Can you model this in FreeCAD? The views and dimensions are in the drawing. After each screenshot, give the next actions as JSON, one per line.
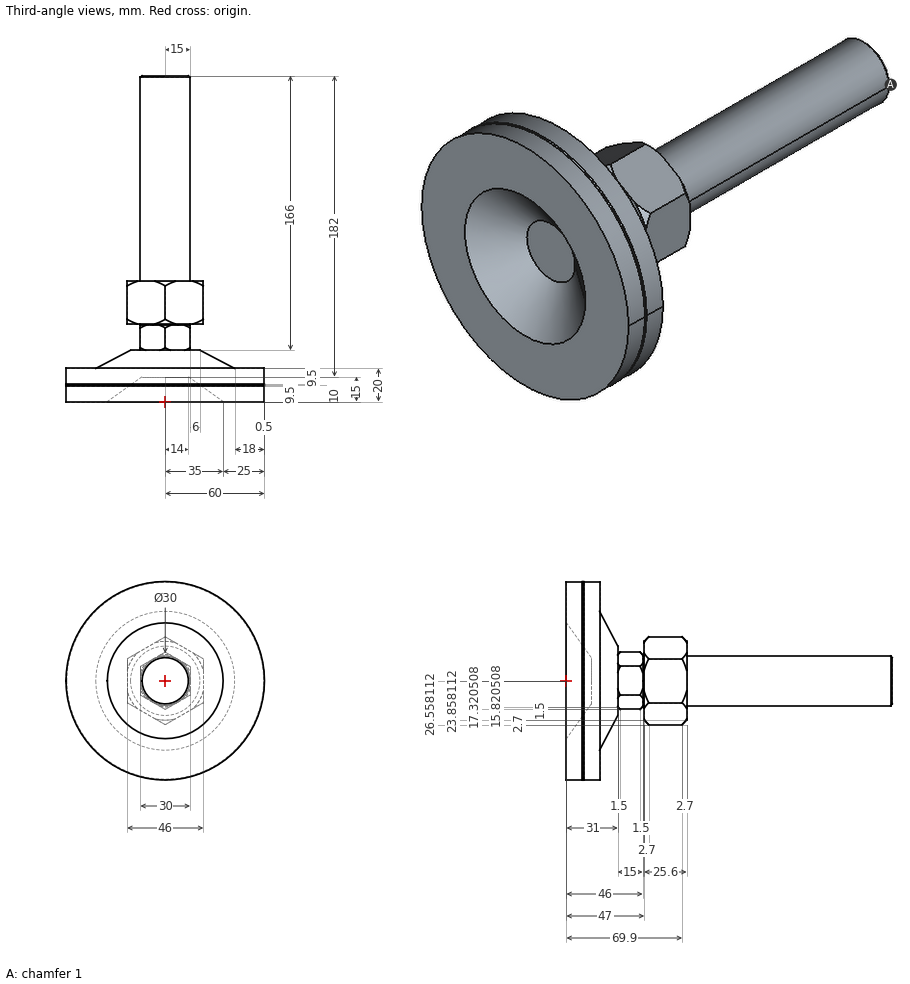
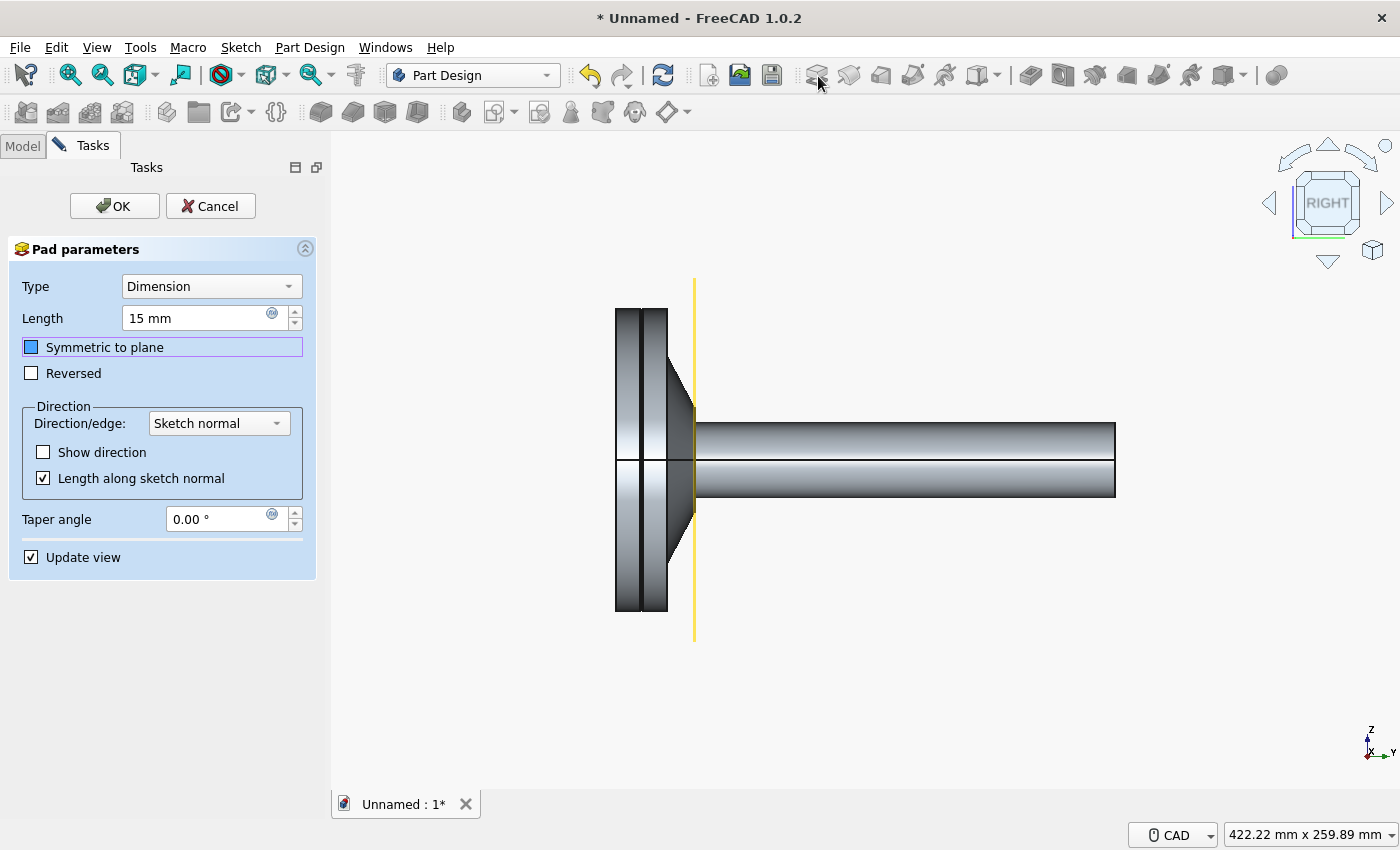
{"action": "left_click", "coordinate": [30, 373]}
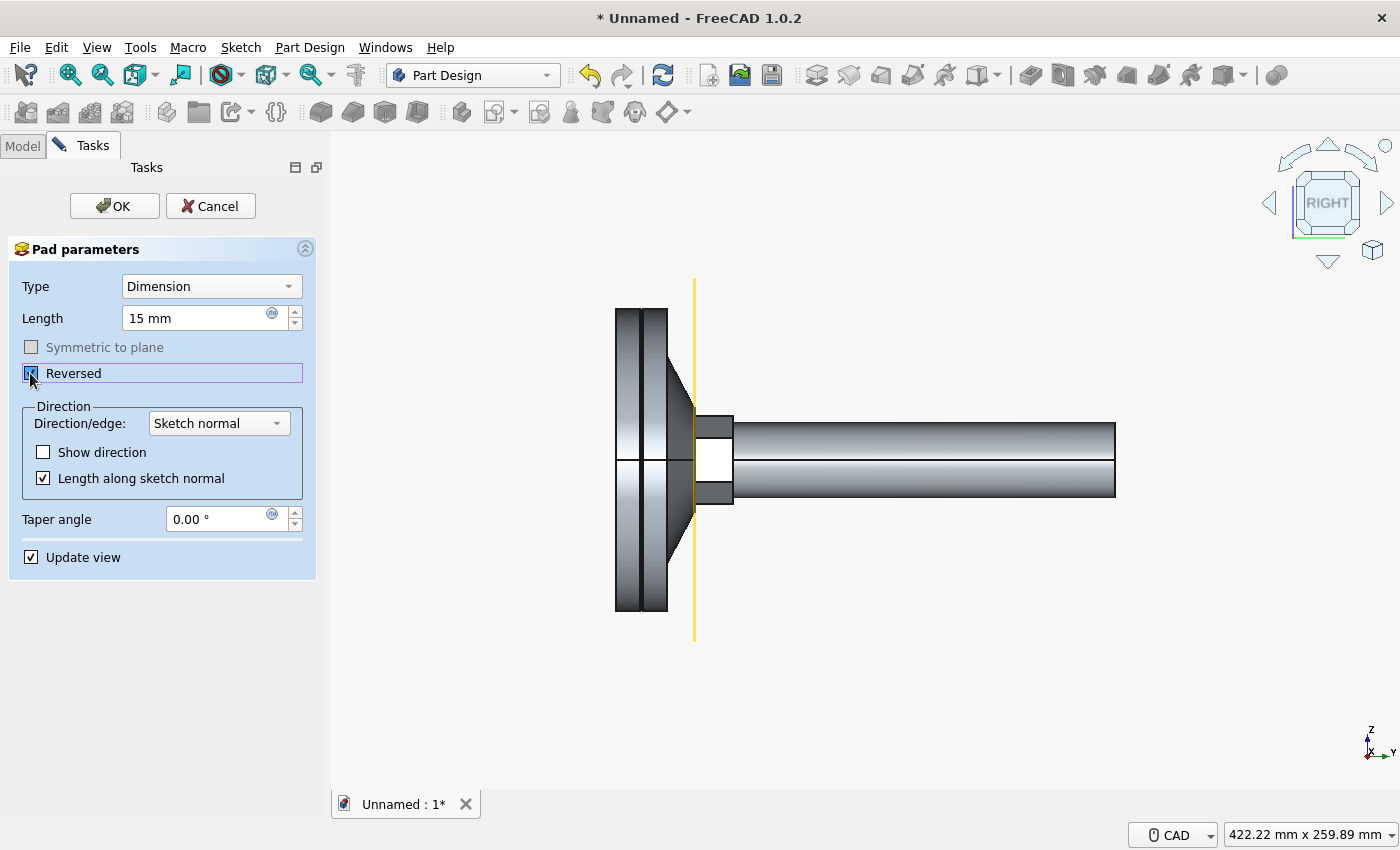
{"action": "left_click", "coordinate": [115, 206]}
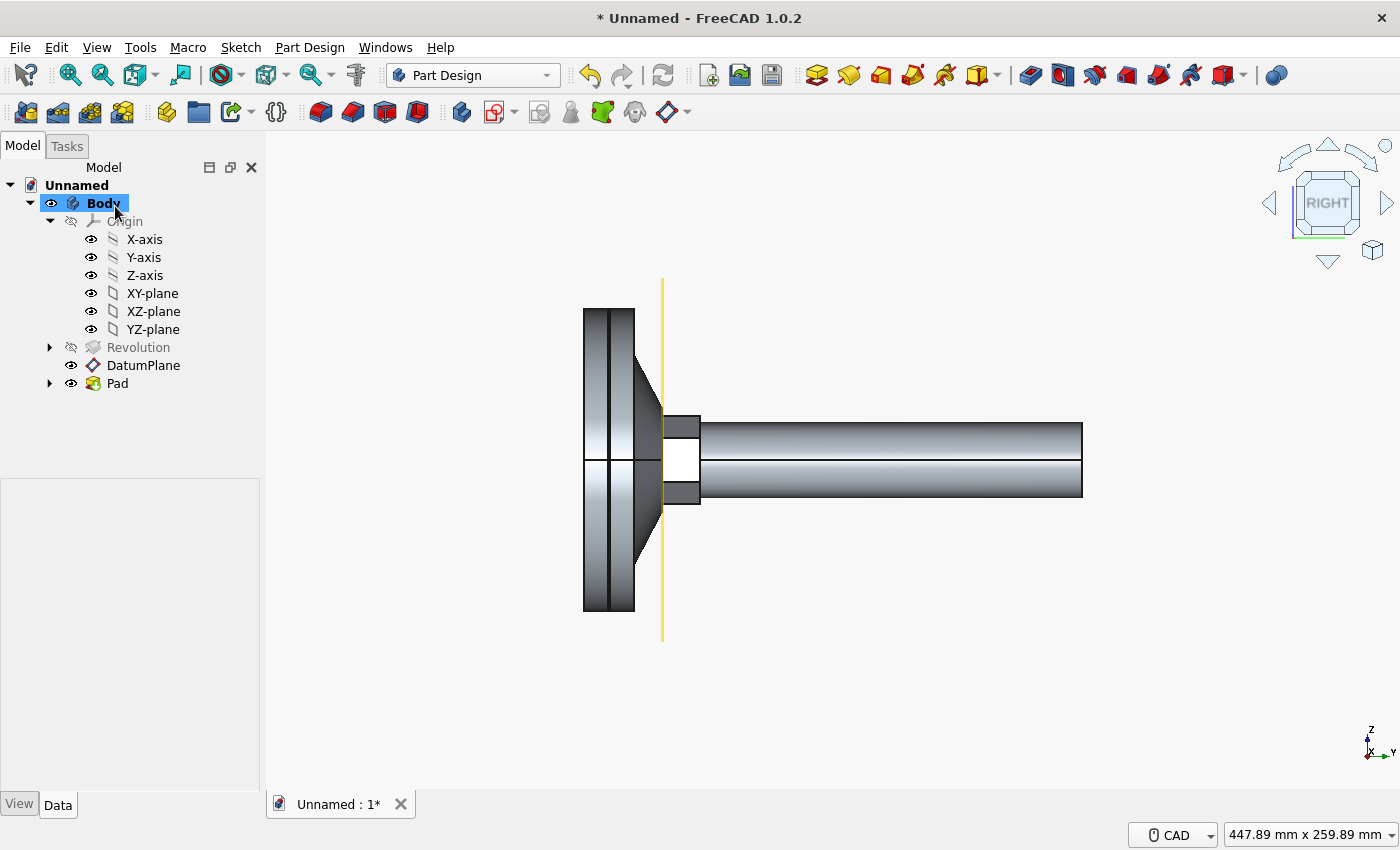
{"action": "left_click", "coordinate": [116, 365]}
{"action": "key", "text": "space"}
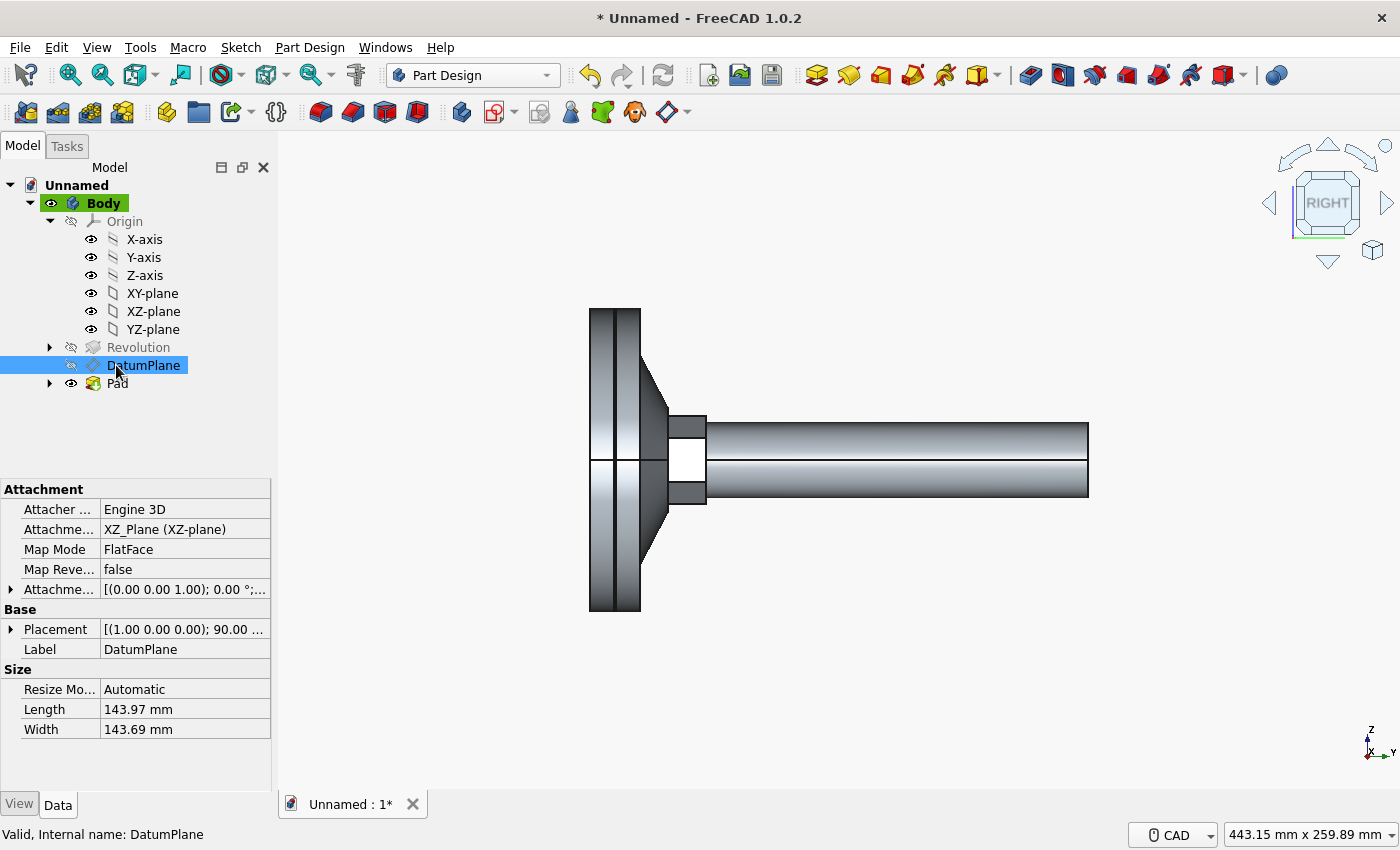
{"action": "left_click", "coordinate": [318, 749]}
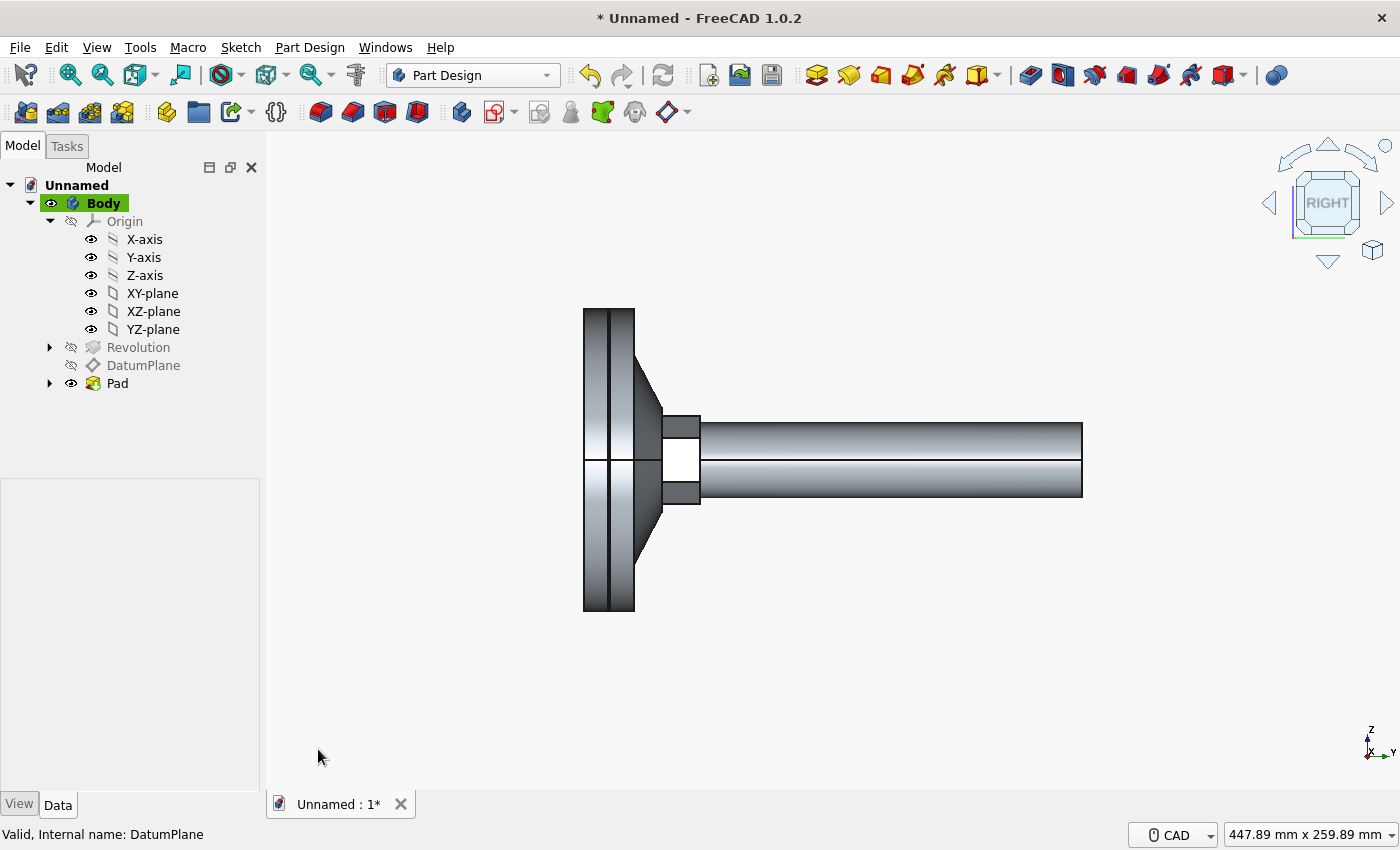
{"action": "left_click", "coordinate": [494, 112]}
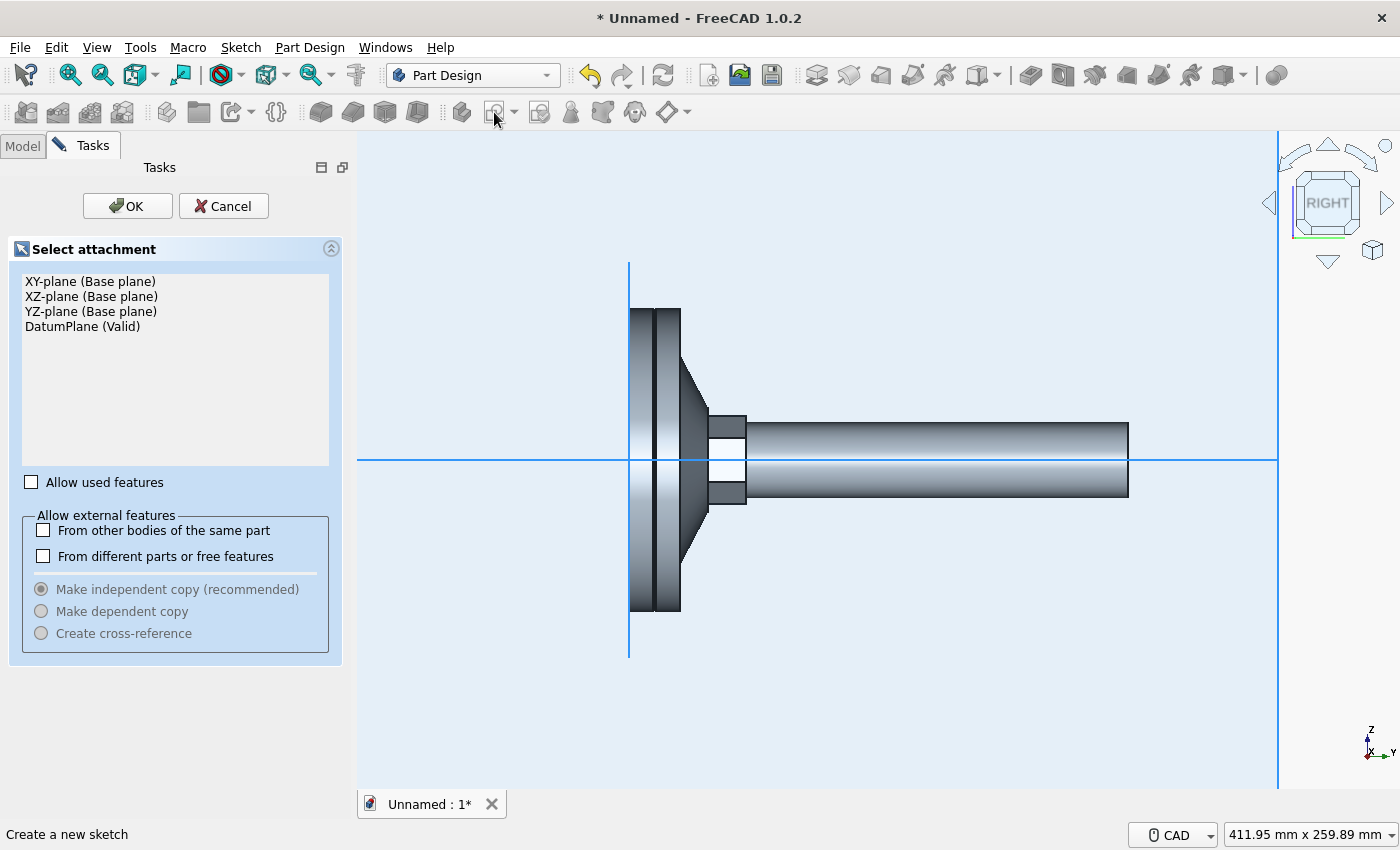
{"action": "left_click", "coordinate": [82, 312]}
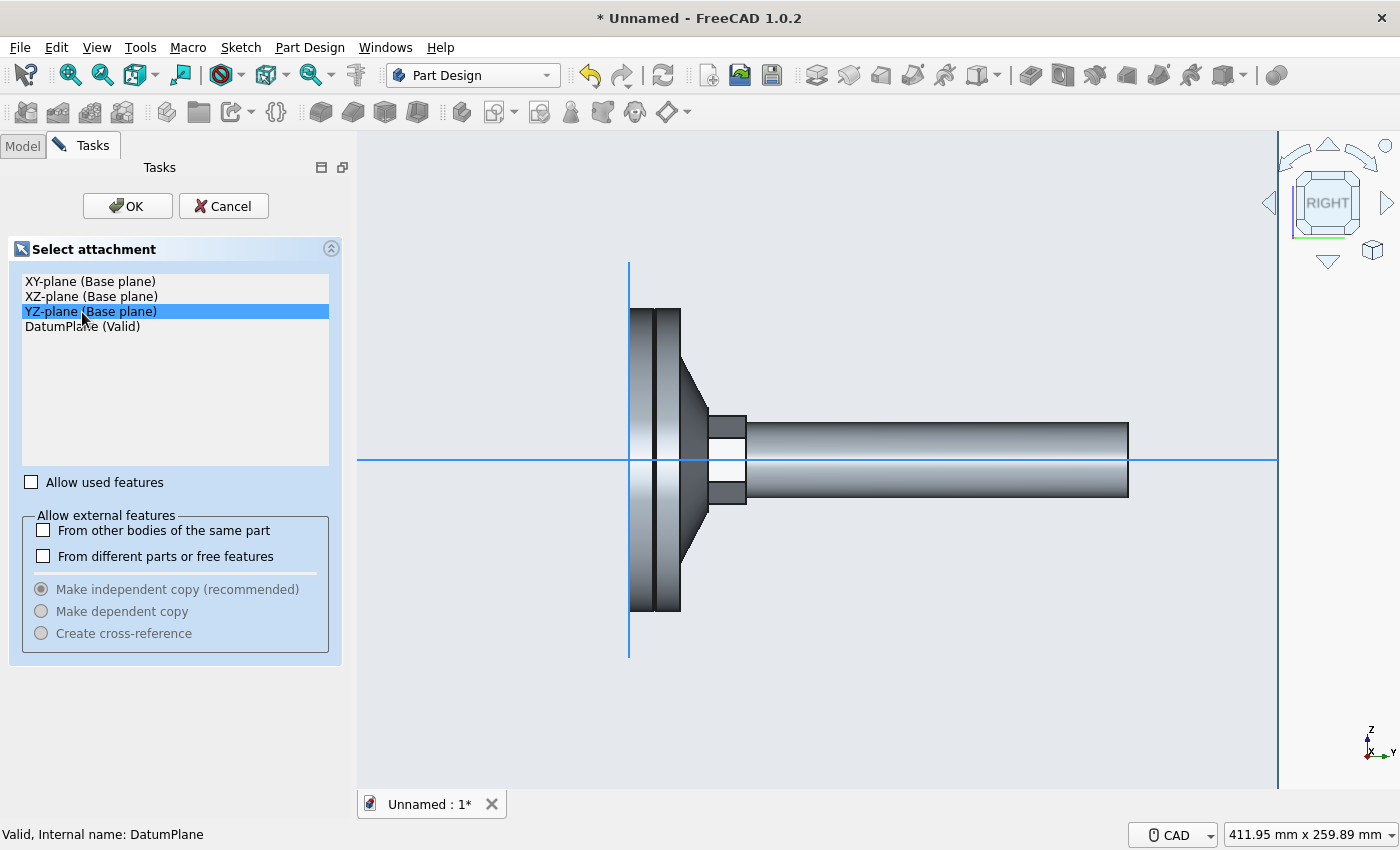
{"action": "left_click", "coordinate": [128, 206]}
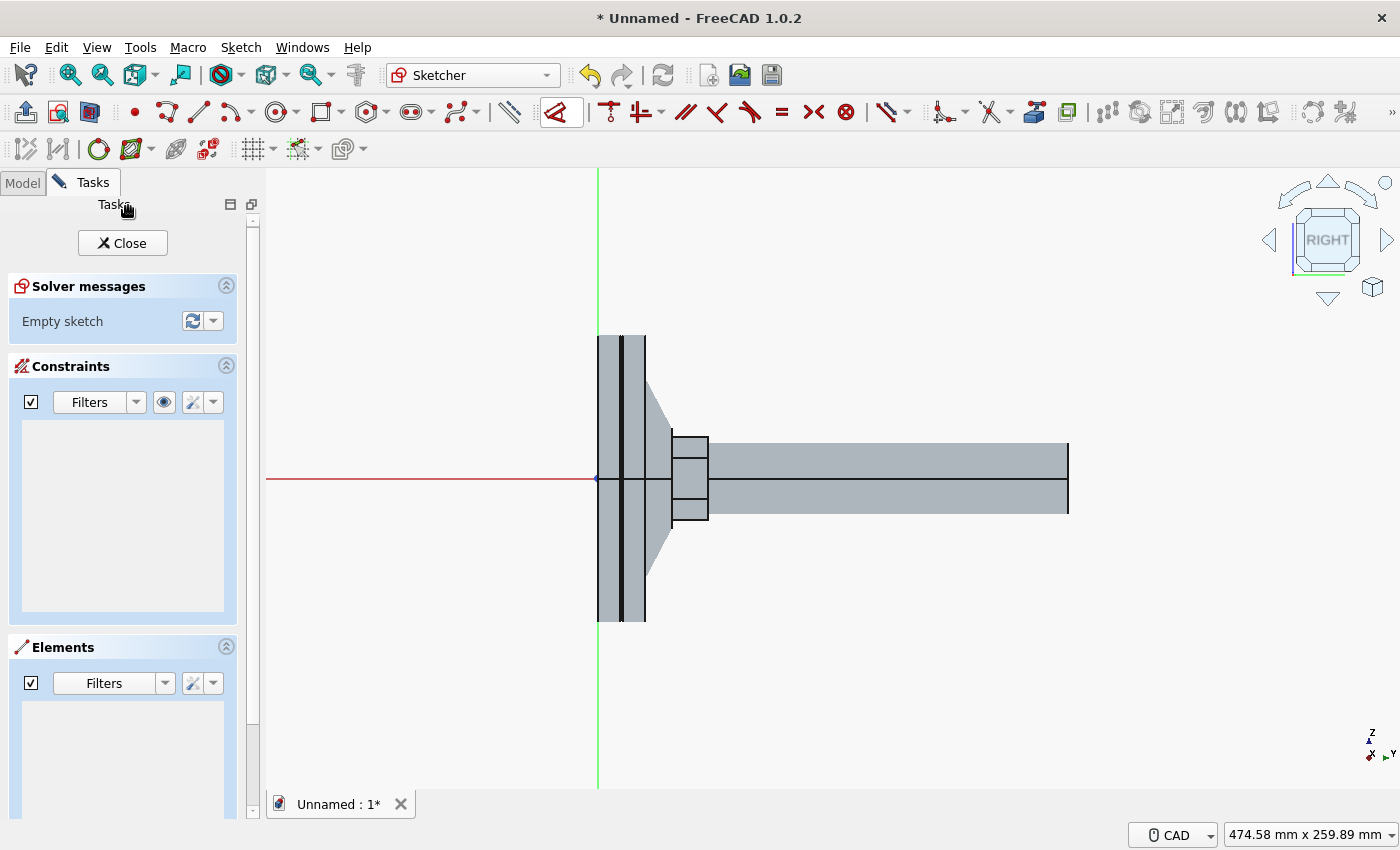
{"action": "key", "text": "q s"}